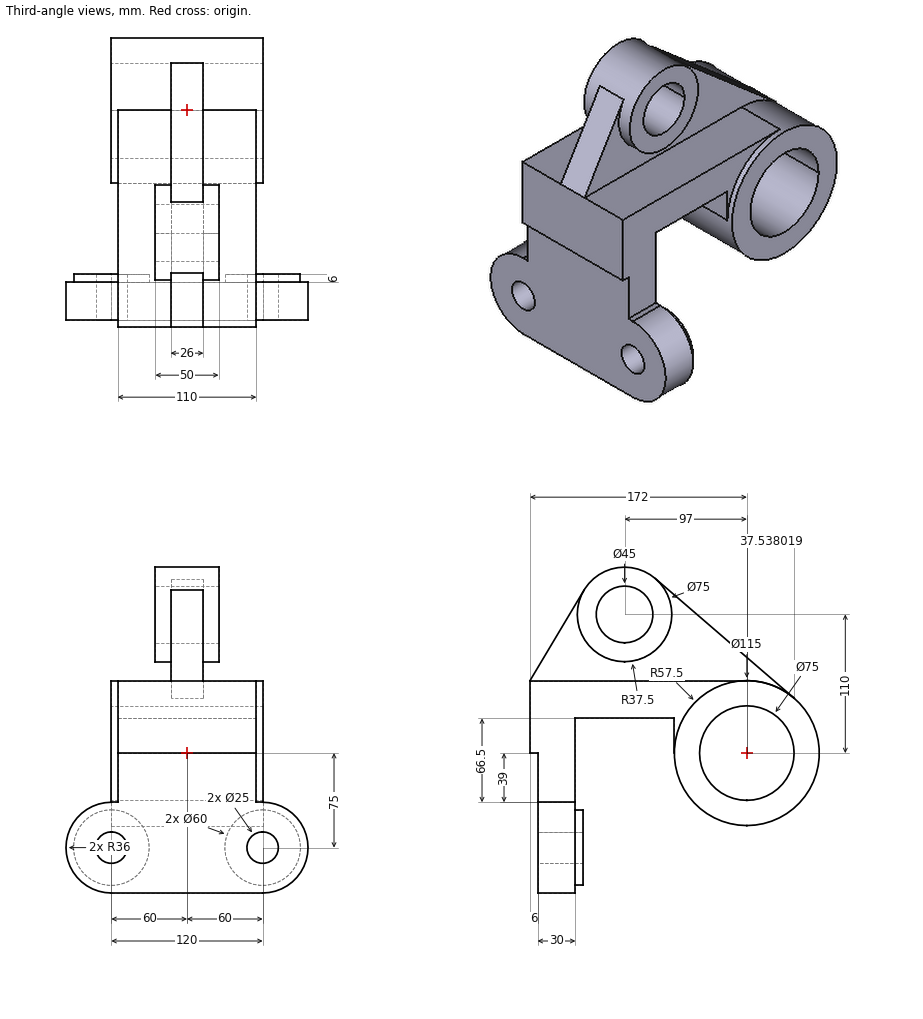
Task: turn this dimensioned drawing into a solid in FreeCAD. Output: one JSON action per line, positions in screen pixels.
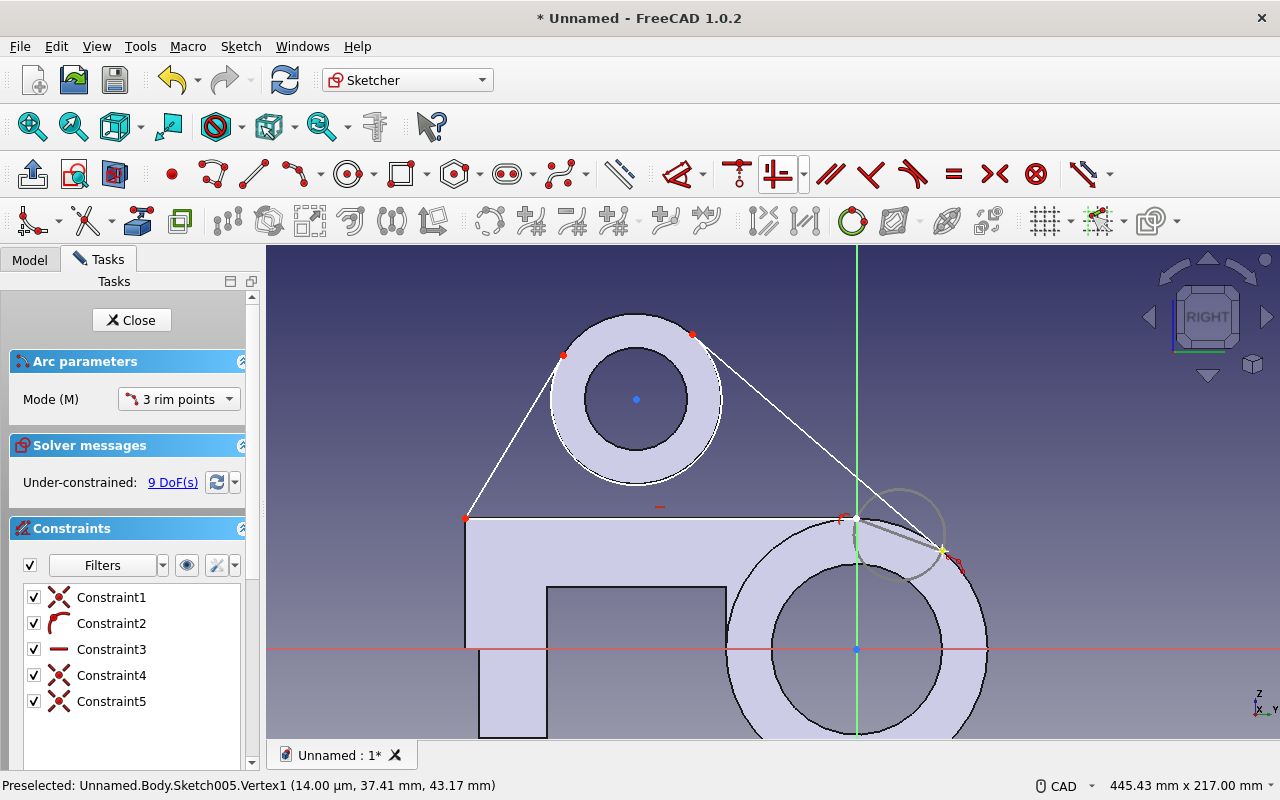
{"action": "scroll", "coordinate": [902, 527], "scroll_direction": "up", "scroll_amount": 4}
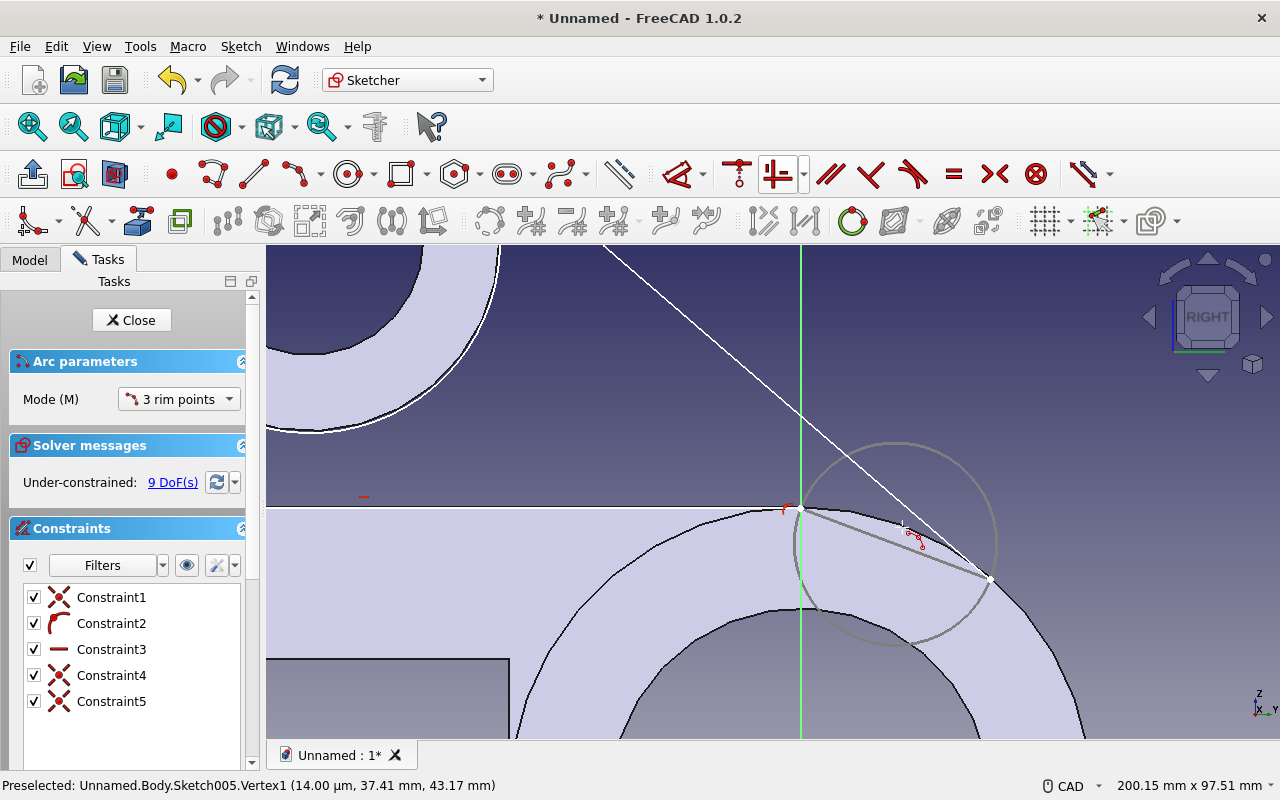
{"action": "left_click", "coordinate": [902, 525]}
{"action": "key", "text": "Escape"}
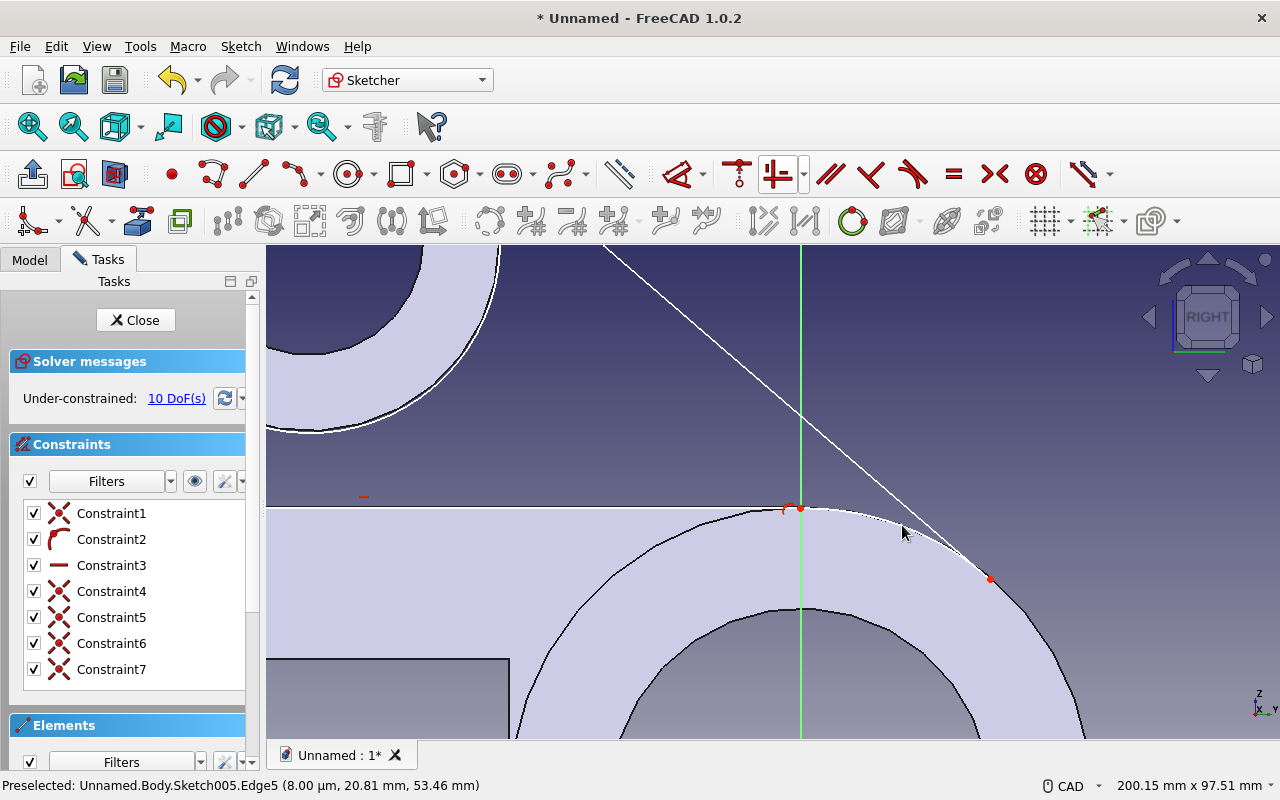
{"action": "left_click", "coordinate": [823, 435]}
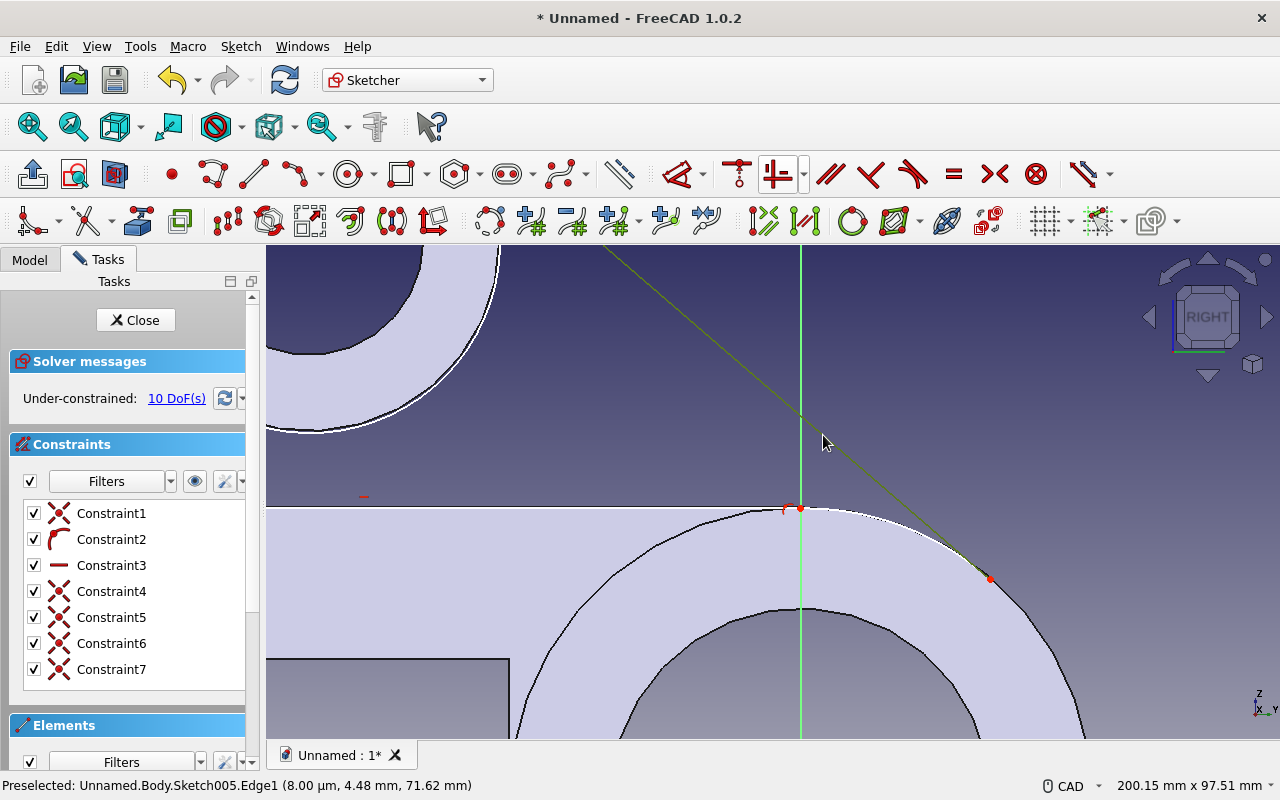
{"action": "left_click", "coordinate": [477, 334]}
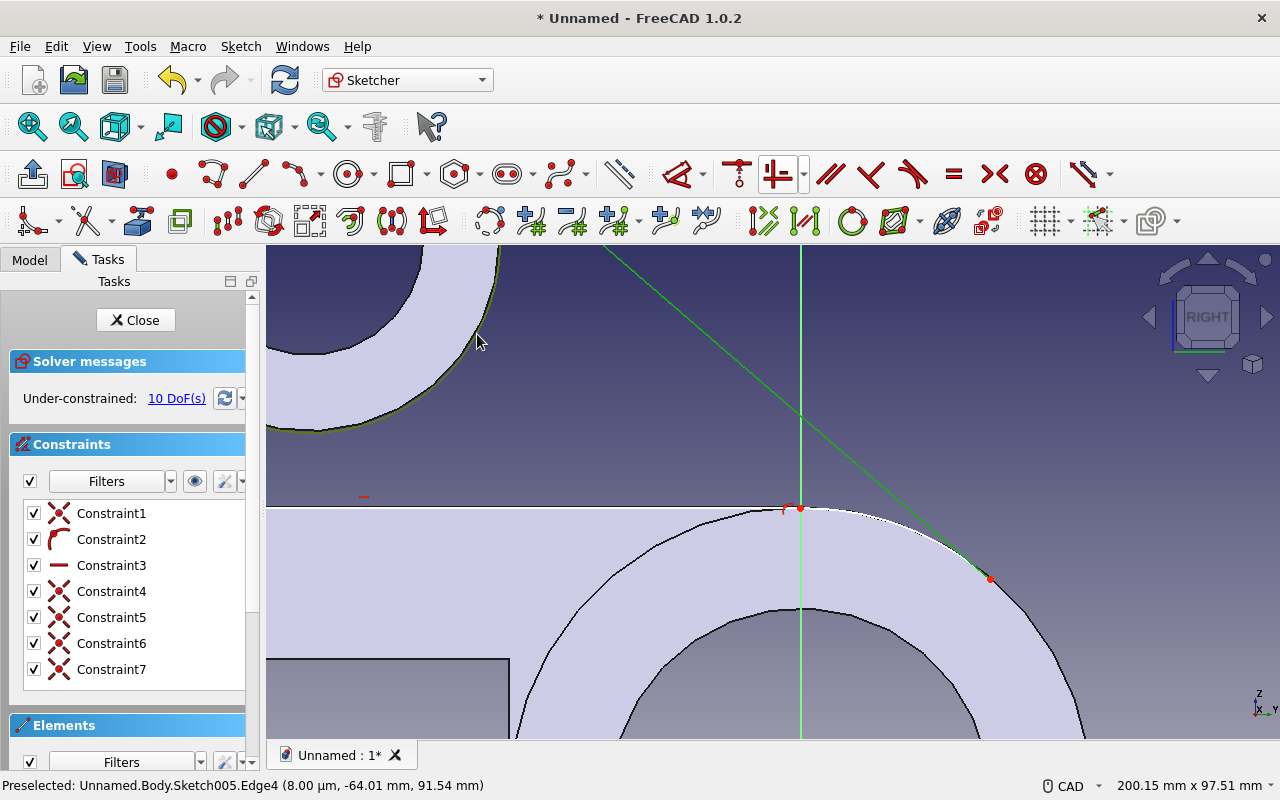
{"action": "key", "text": "t"}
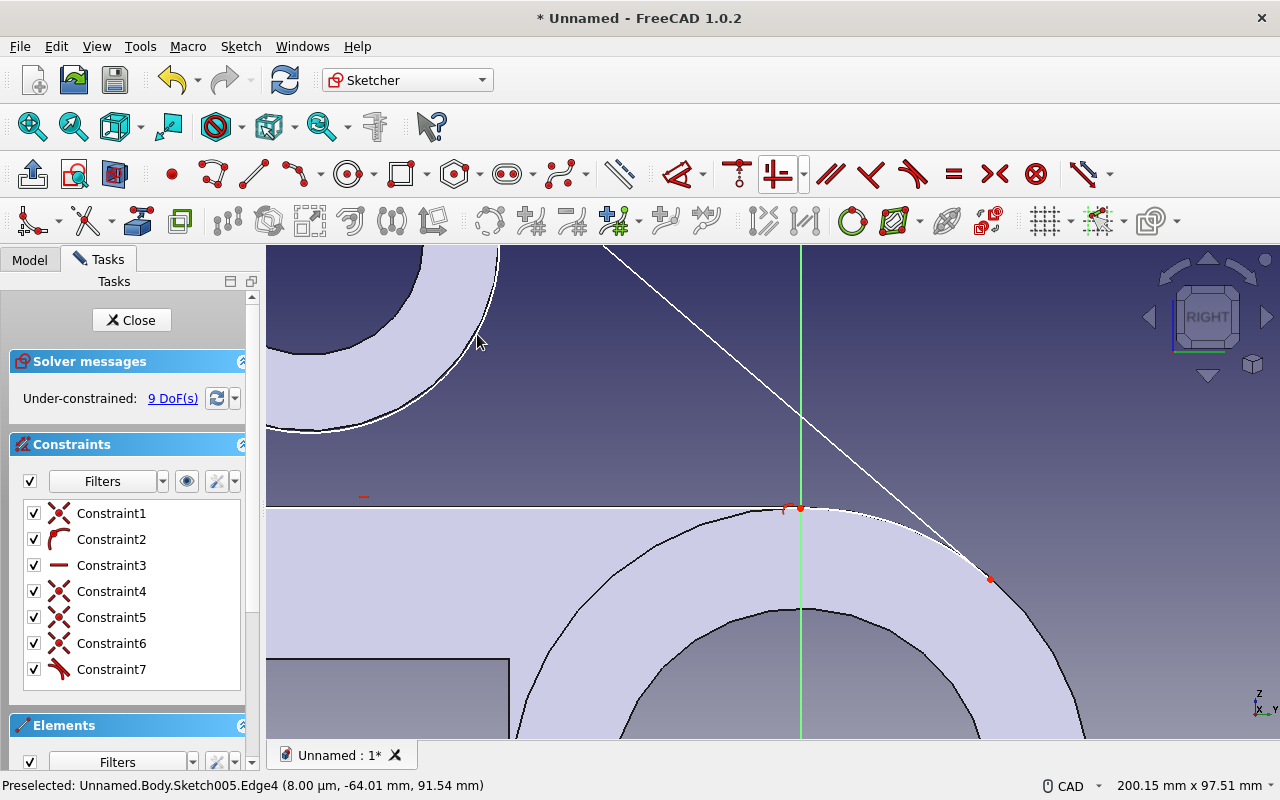
{"action": "scroll", "coordinate": [904, 528], "scroll_direction": "down", "scroll_amount": 4}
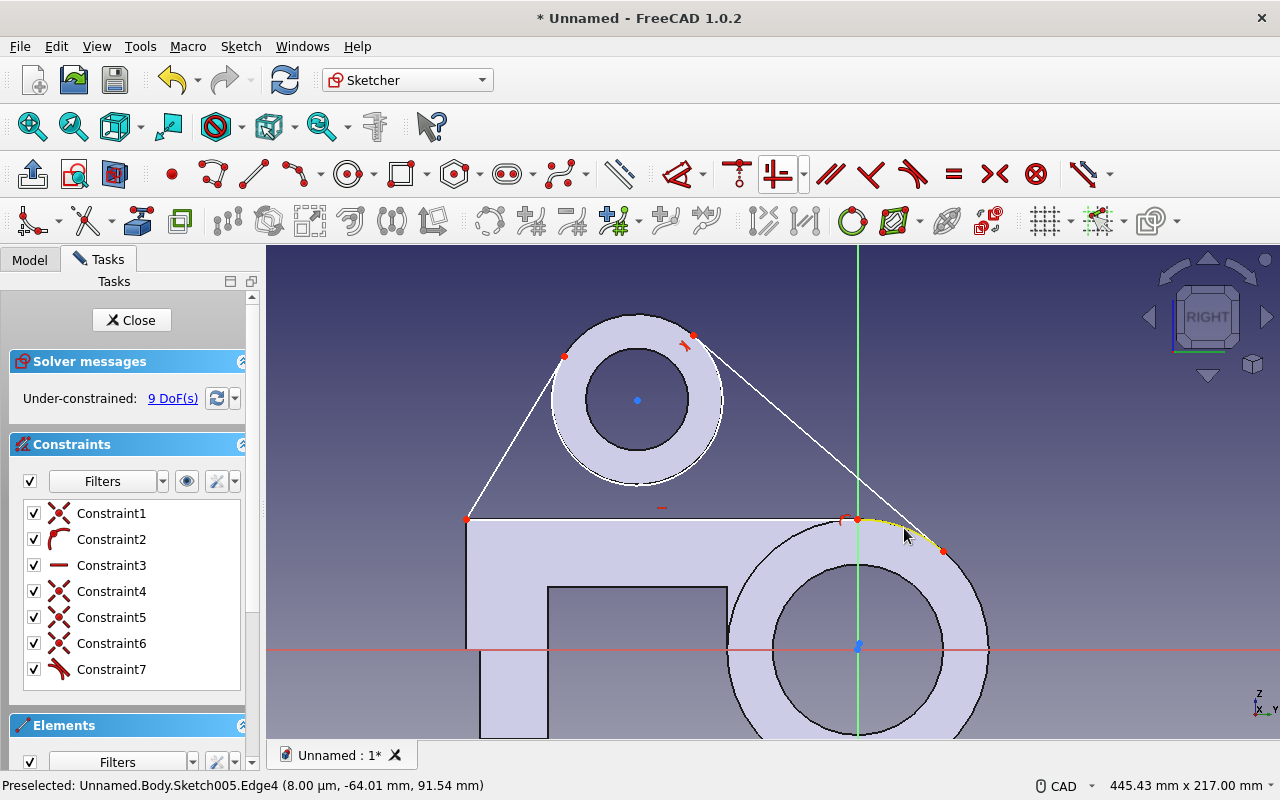
{"action": "left_click", "coordinate": [535, 405]}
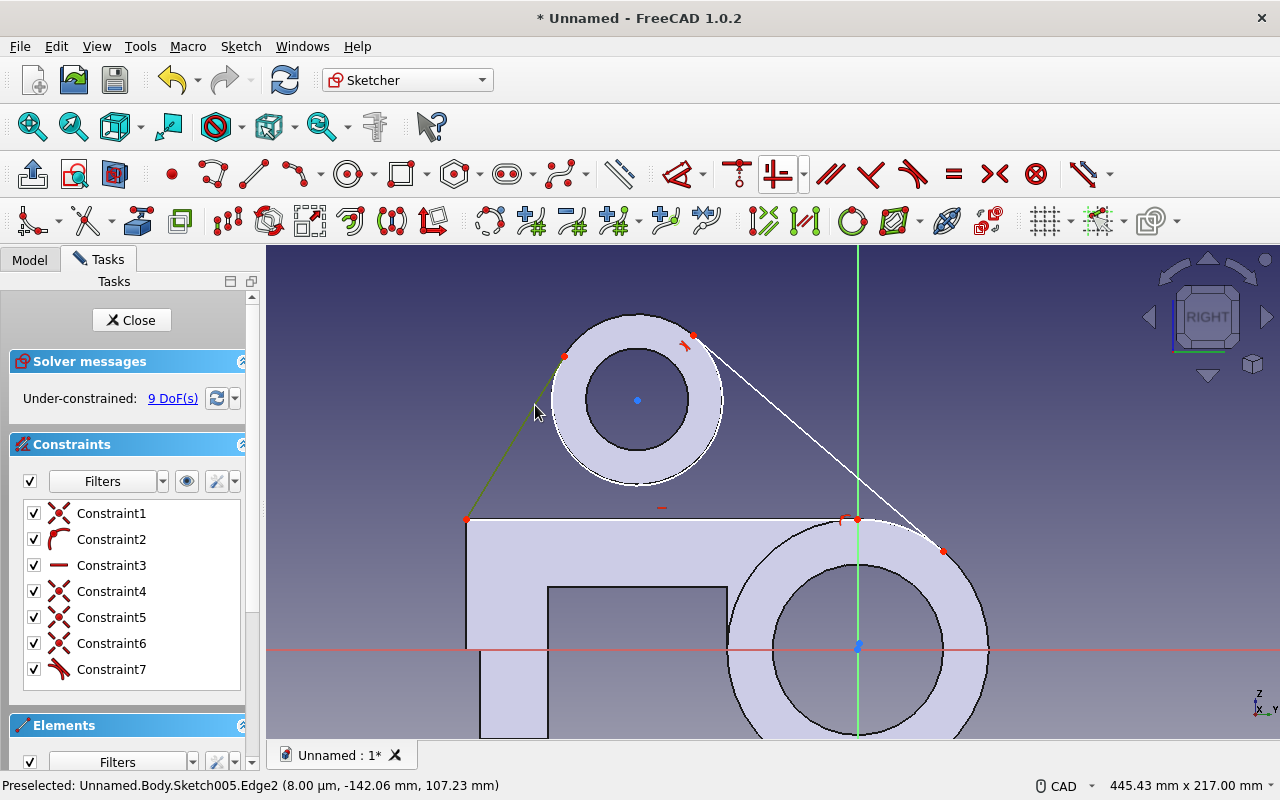
{"action": "left_click", "coordinate": [579, 463]}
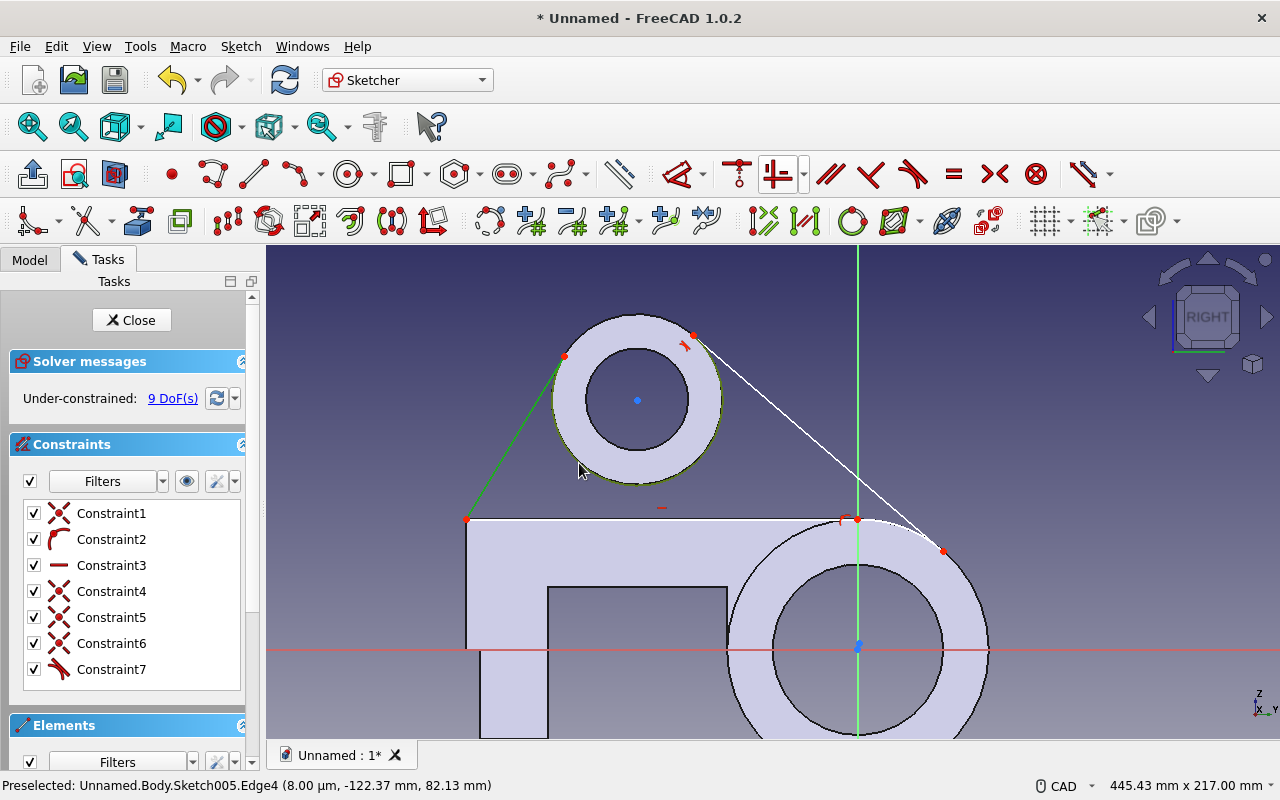
{"action": "left_click", "coordinate": [913, 174]}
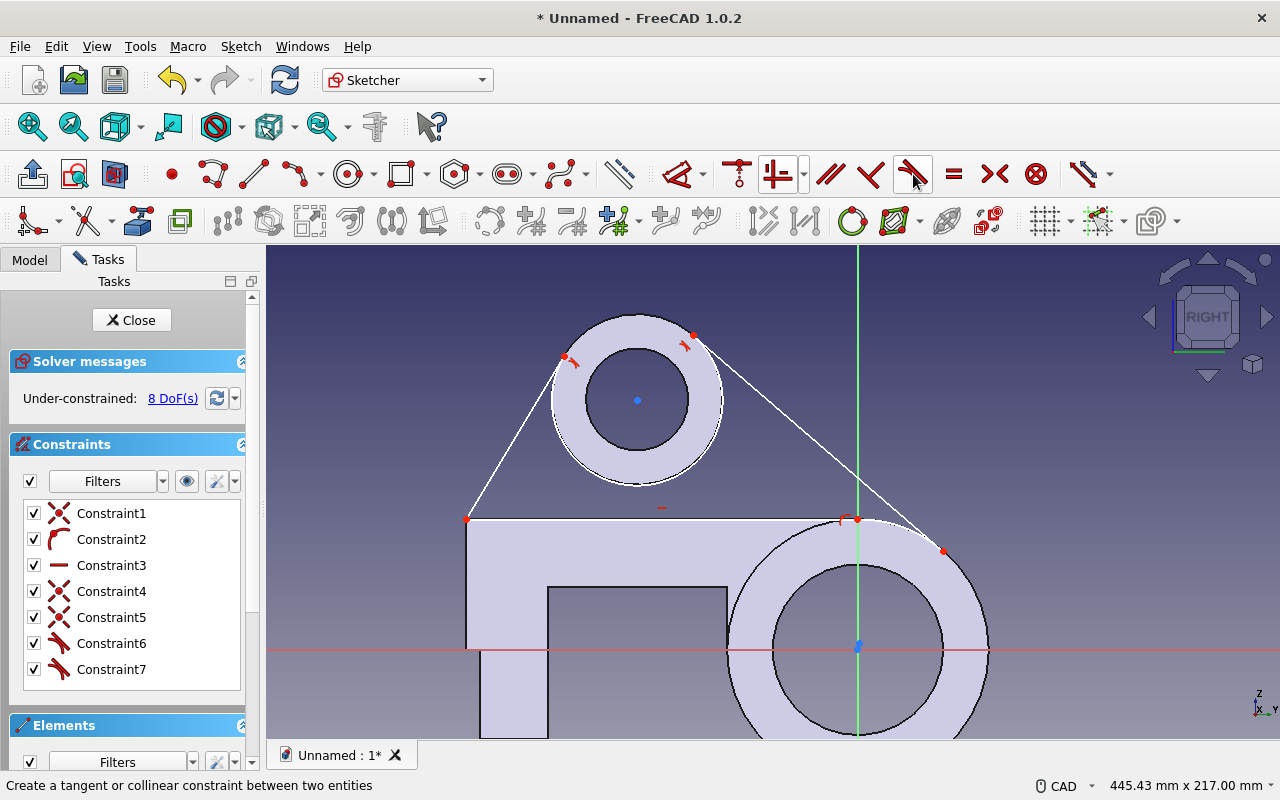
{"action": "left_click_drag", "start_coordinate": [848, 634], "coordinate": [870, 660]}